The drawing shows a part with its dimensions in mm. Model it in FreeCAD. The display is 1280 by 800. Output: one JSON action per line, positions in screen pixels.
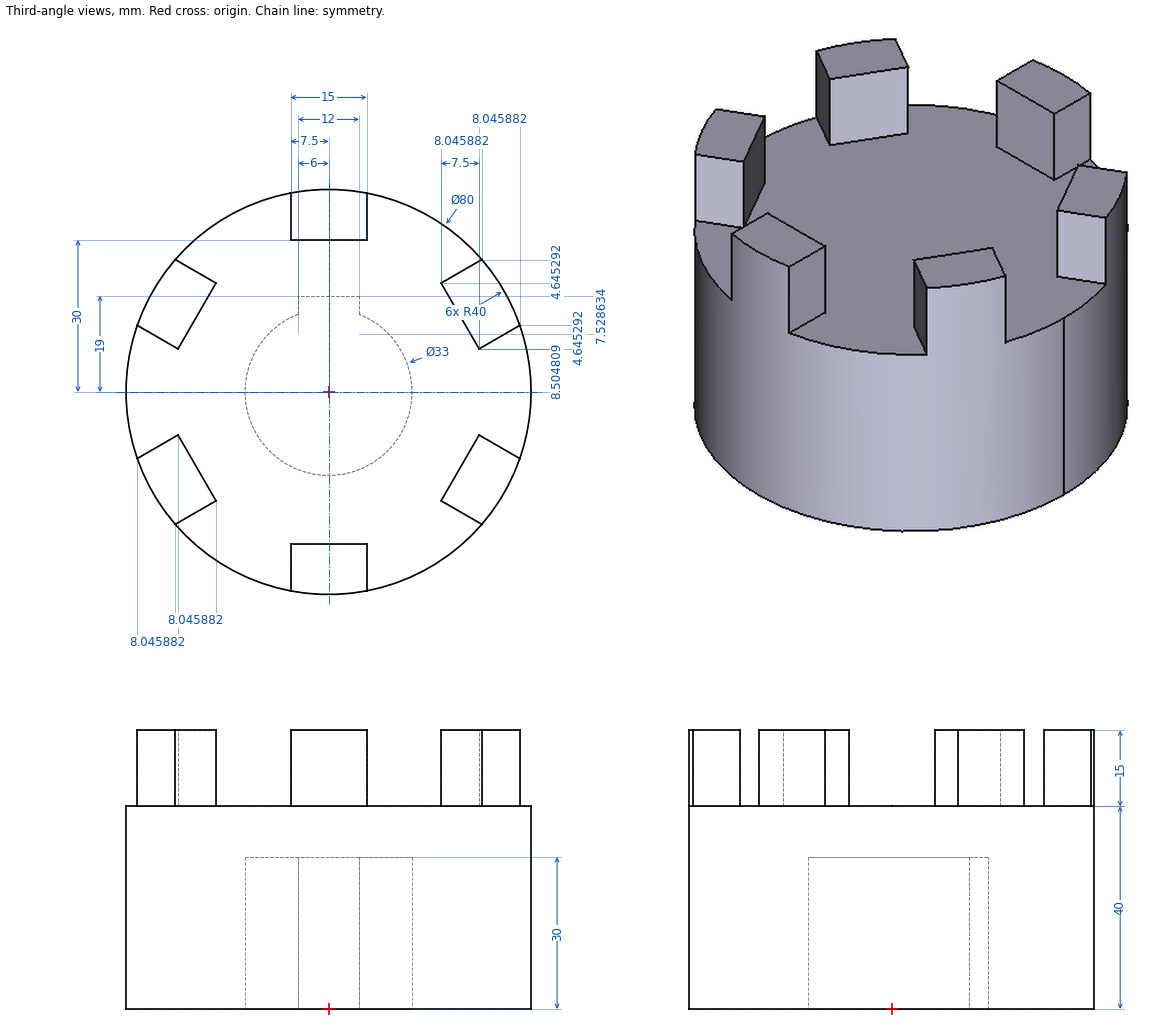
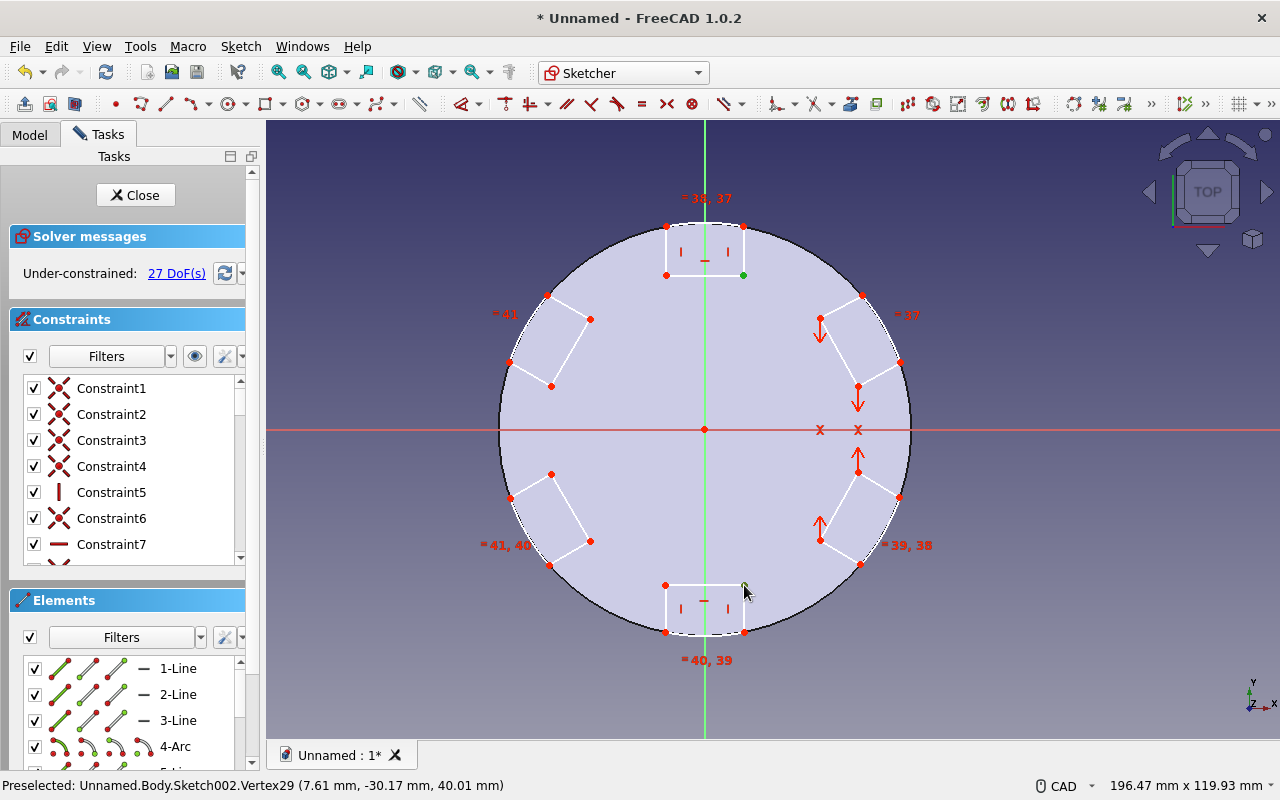
{"action": "left_click", "coordinate": [353, 429]}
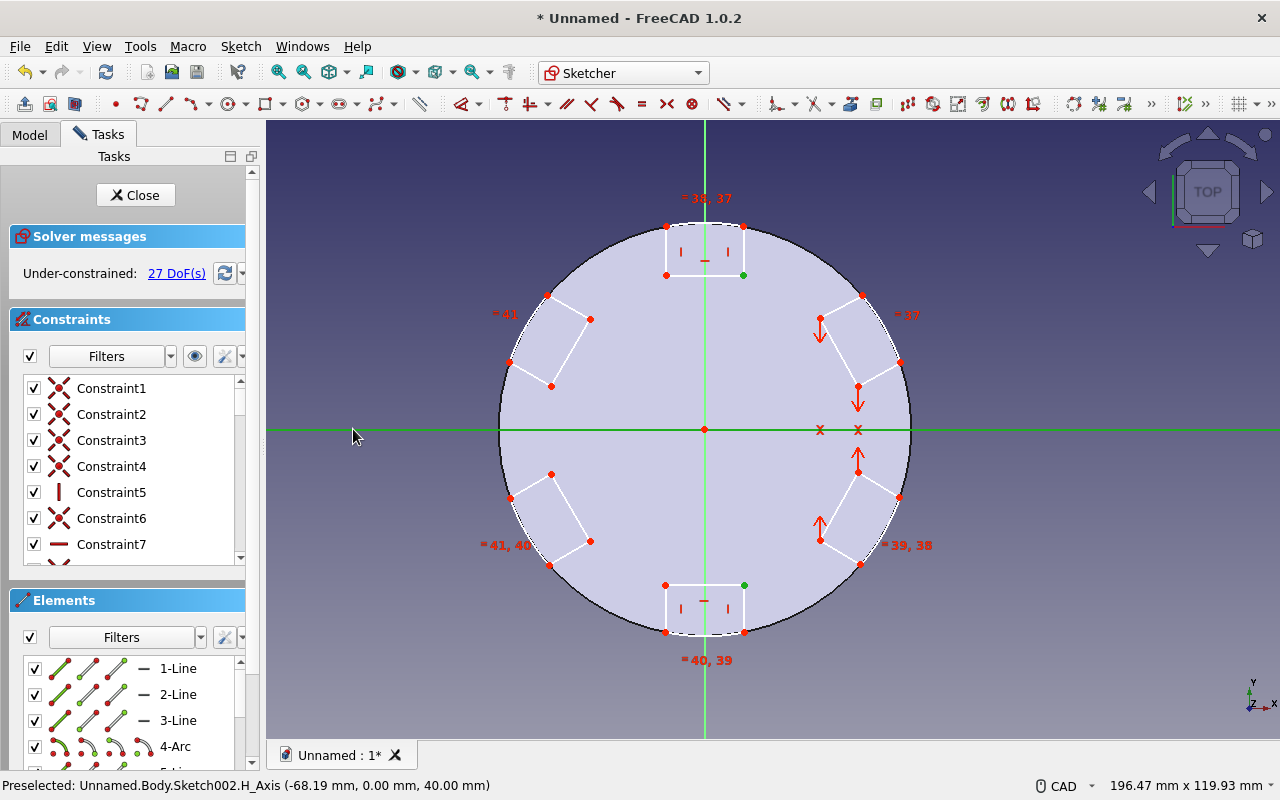
{"action": "key", "text": "s"}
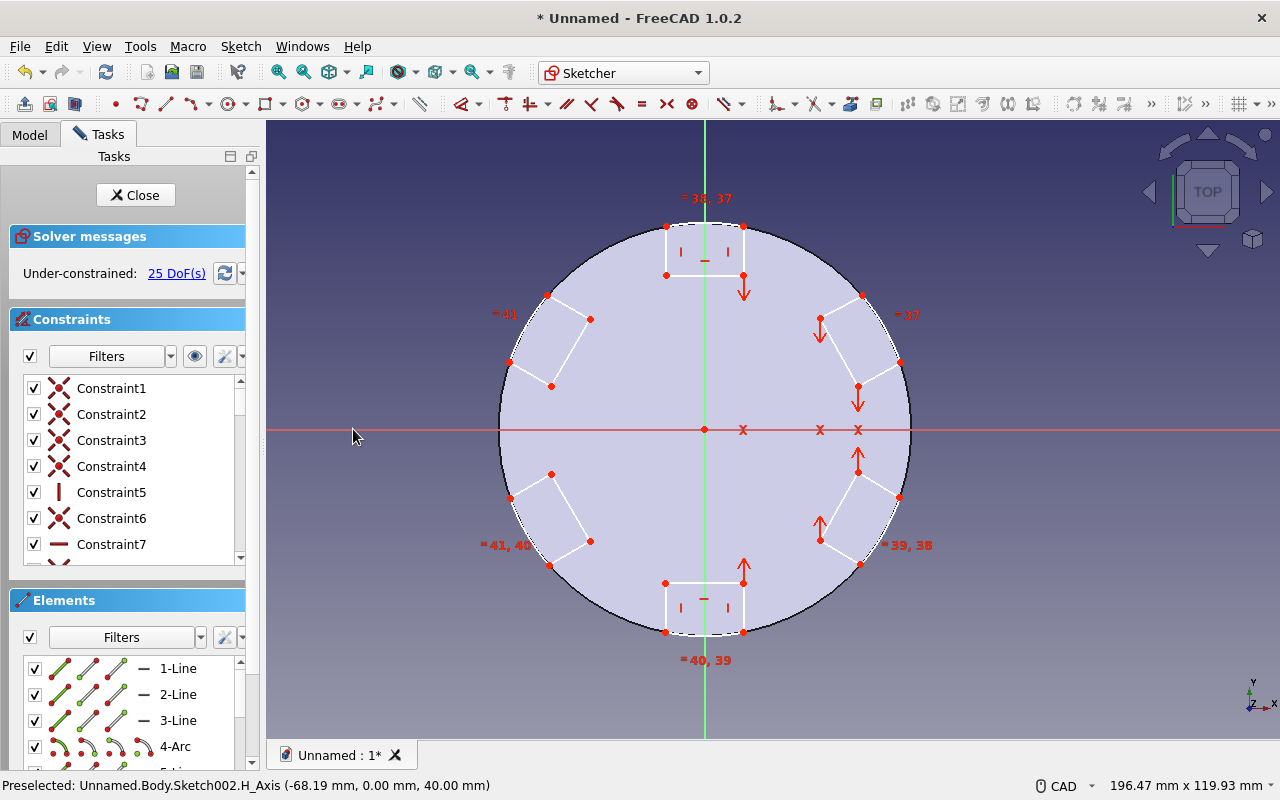
{"action": "left_click", "coordinate": [820, 541]}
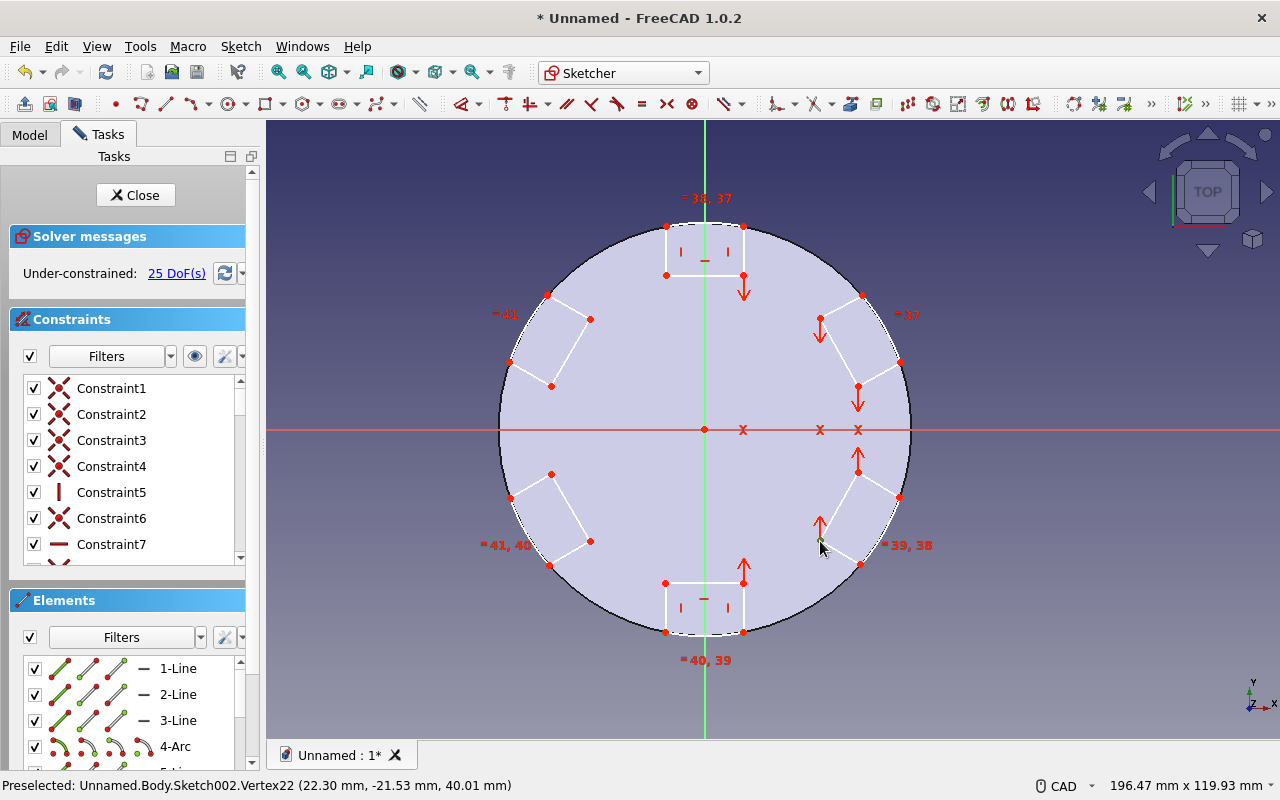
{"action": "left_click", "coordinate": [590, 541]}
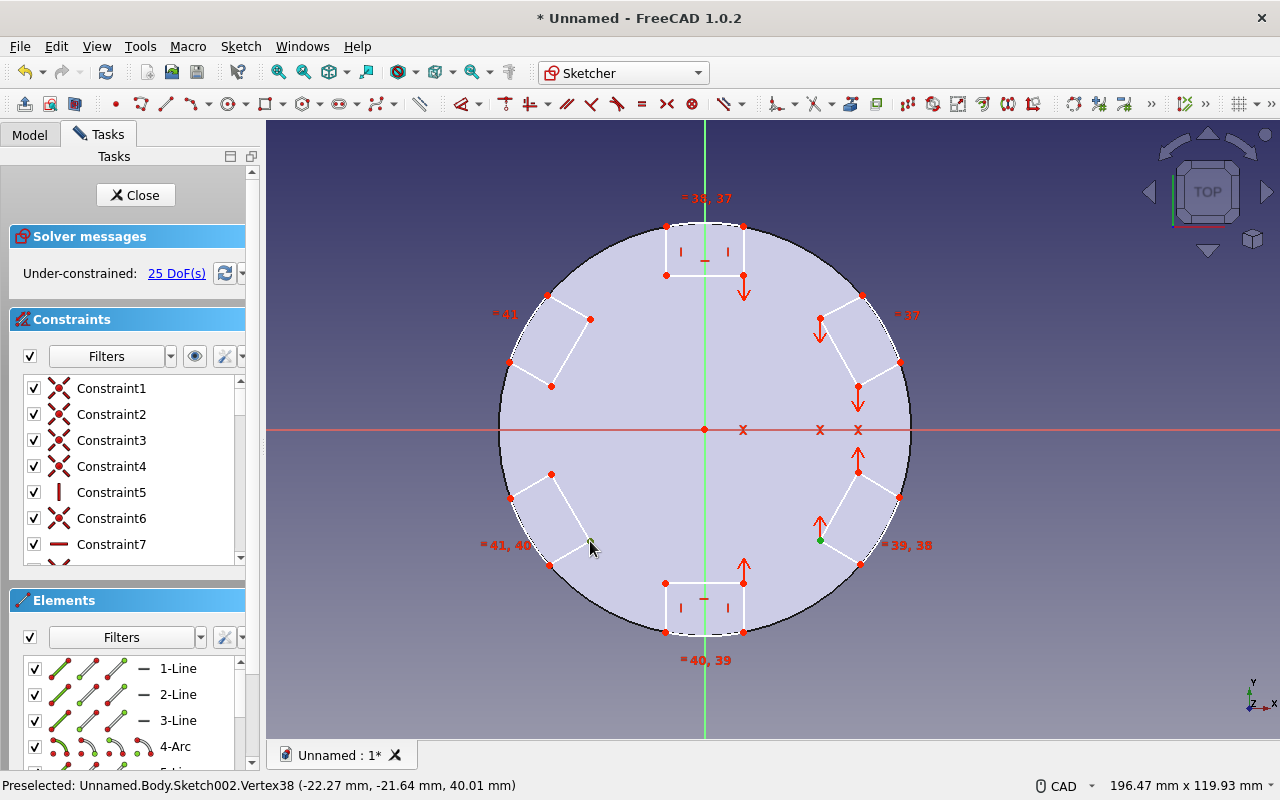
{"action": "left_click", "coordinate": [705, 671]}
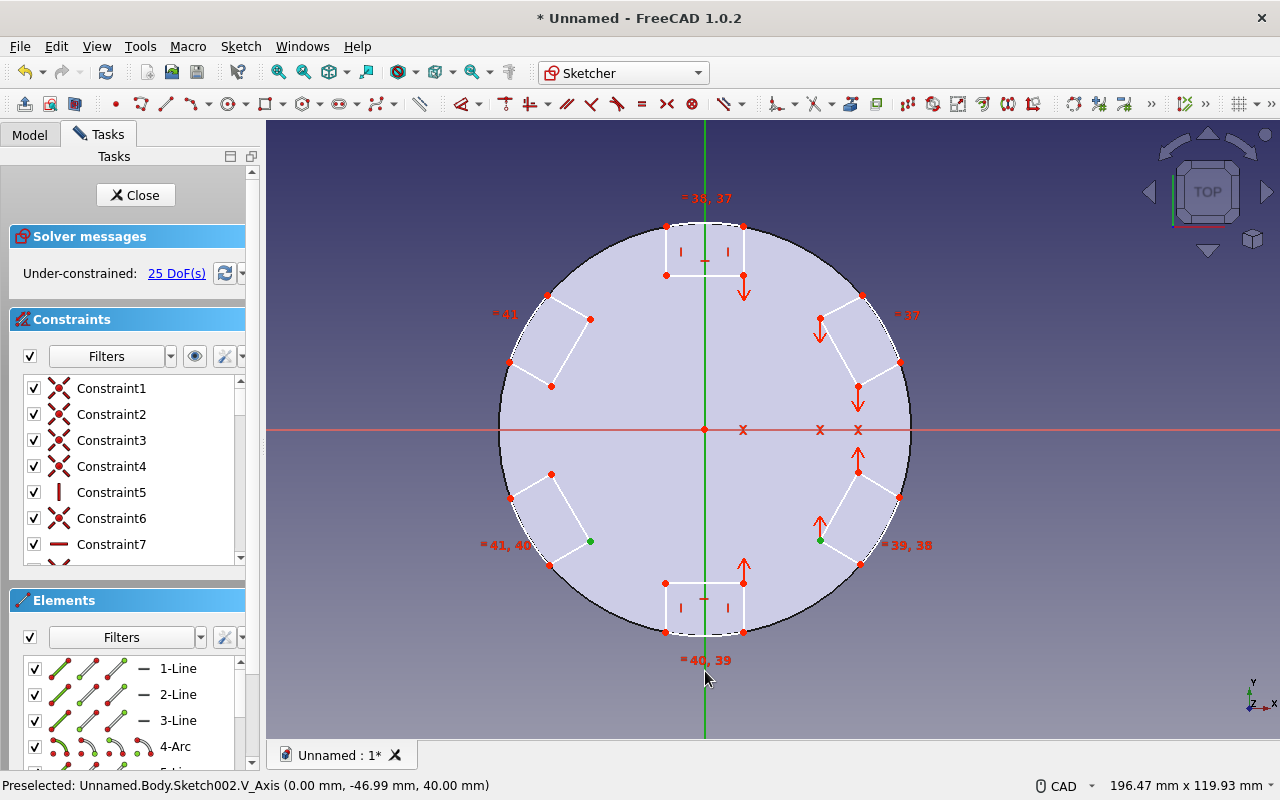
{"action": "key", "text": "s"}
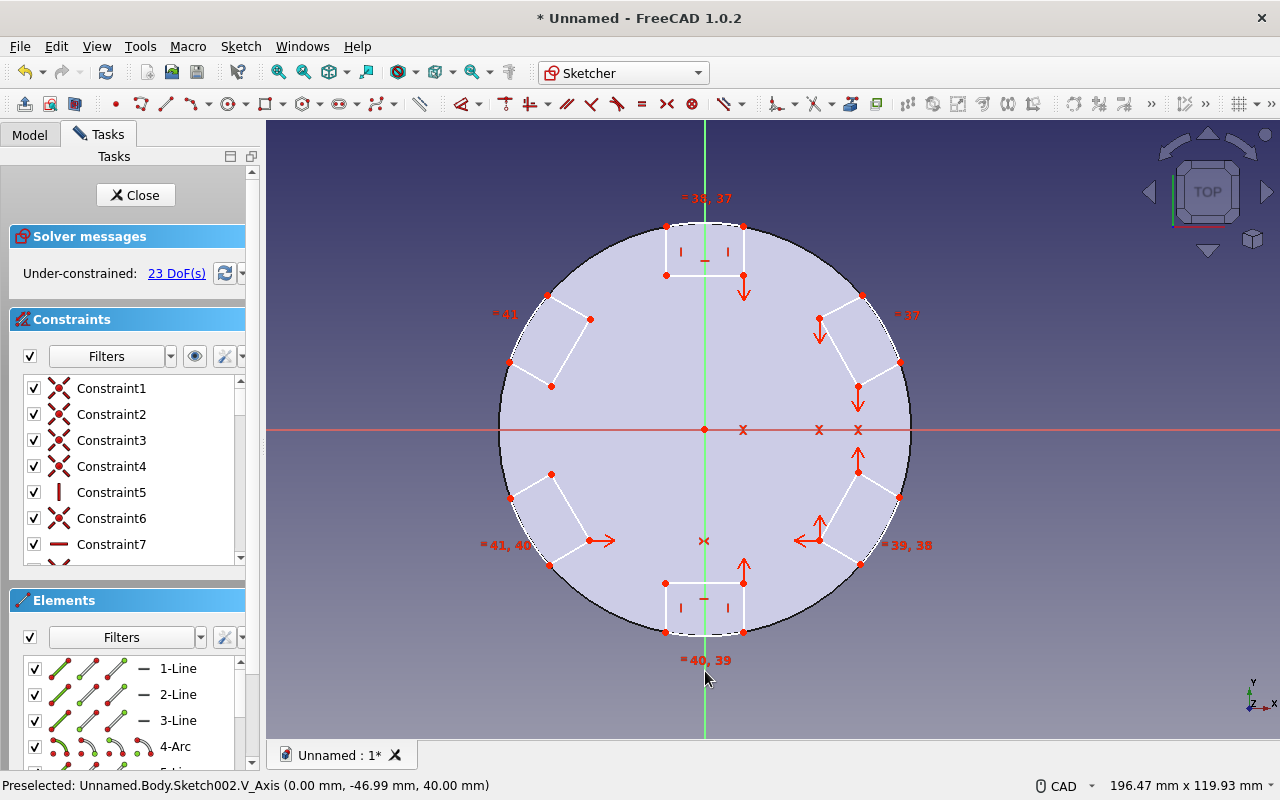
{"action": "left_click", "coordinate": [858, 472]}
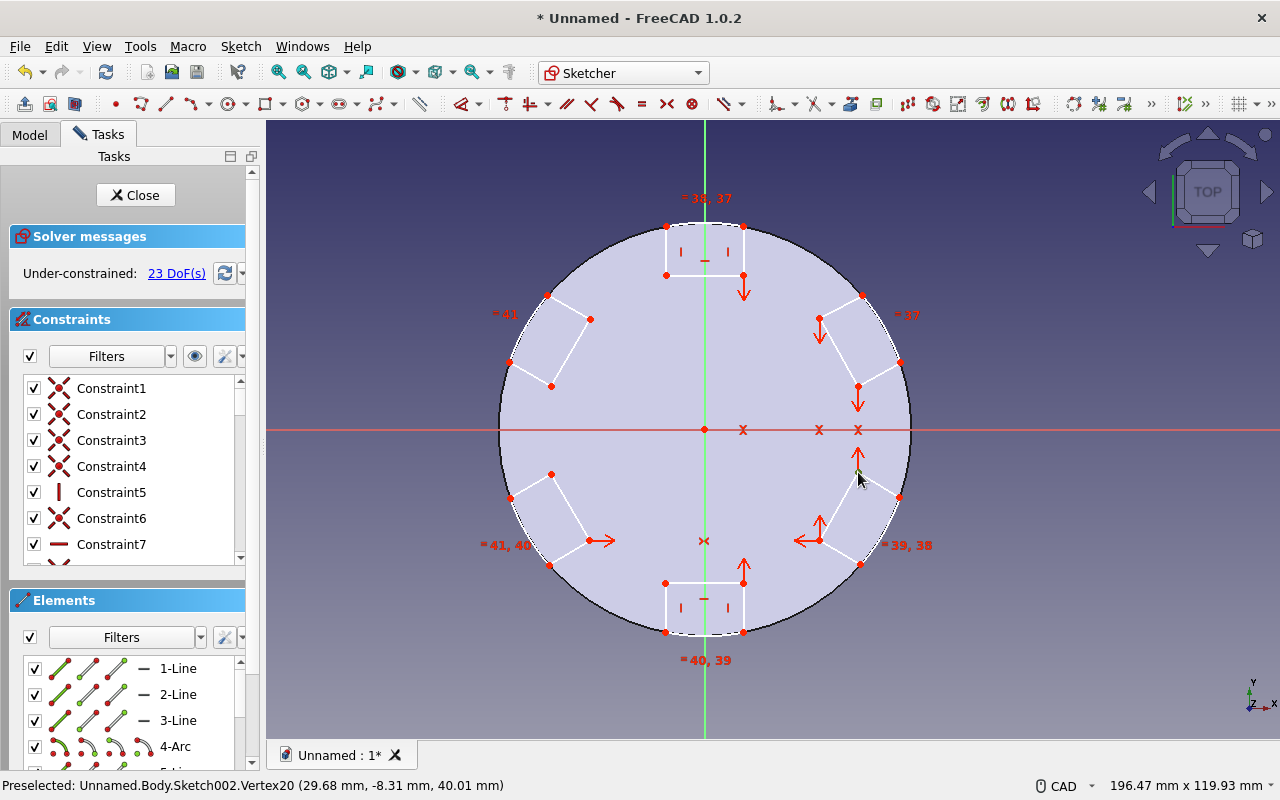
{"action": "left_click", "coordinate": [551, 474]}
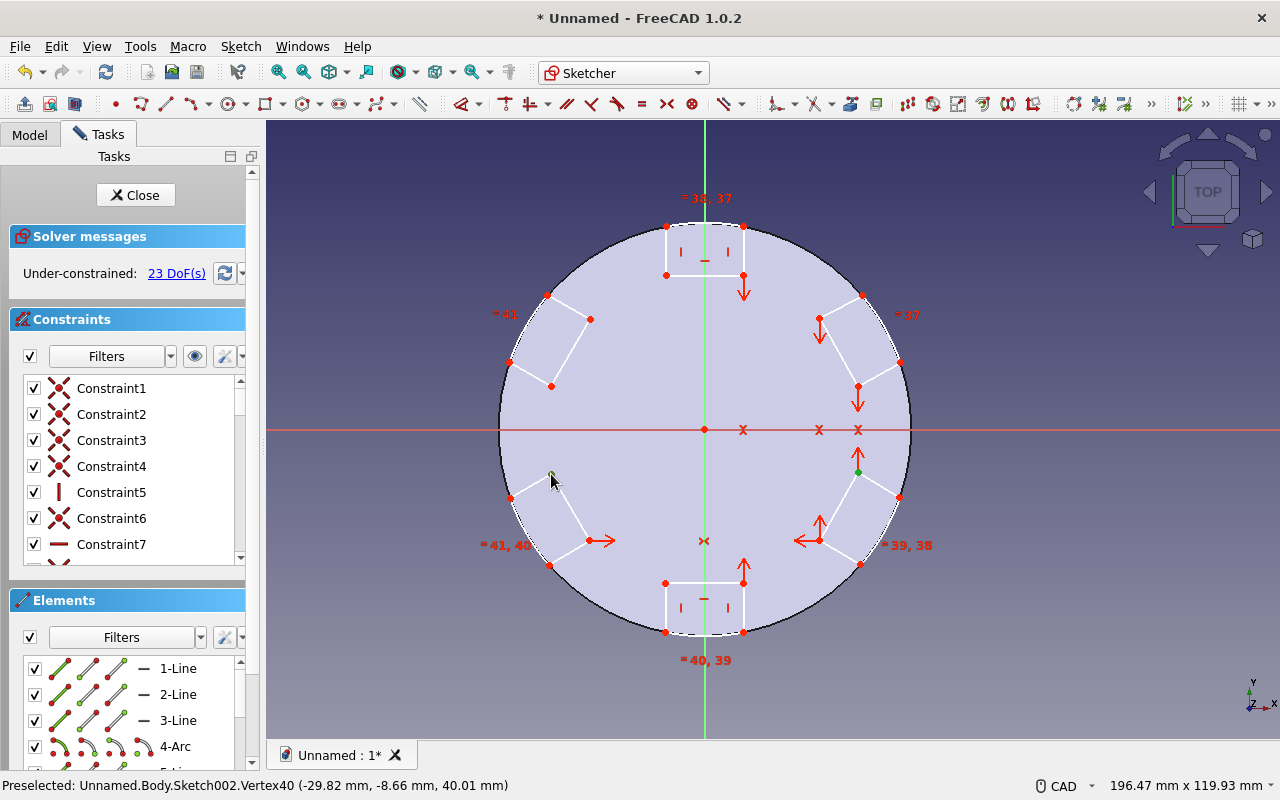
{"action": "left_click", "coordinate": [705, 671]}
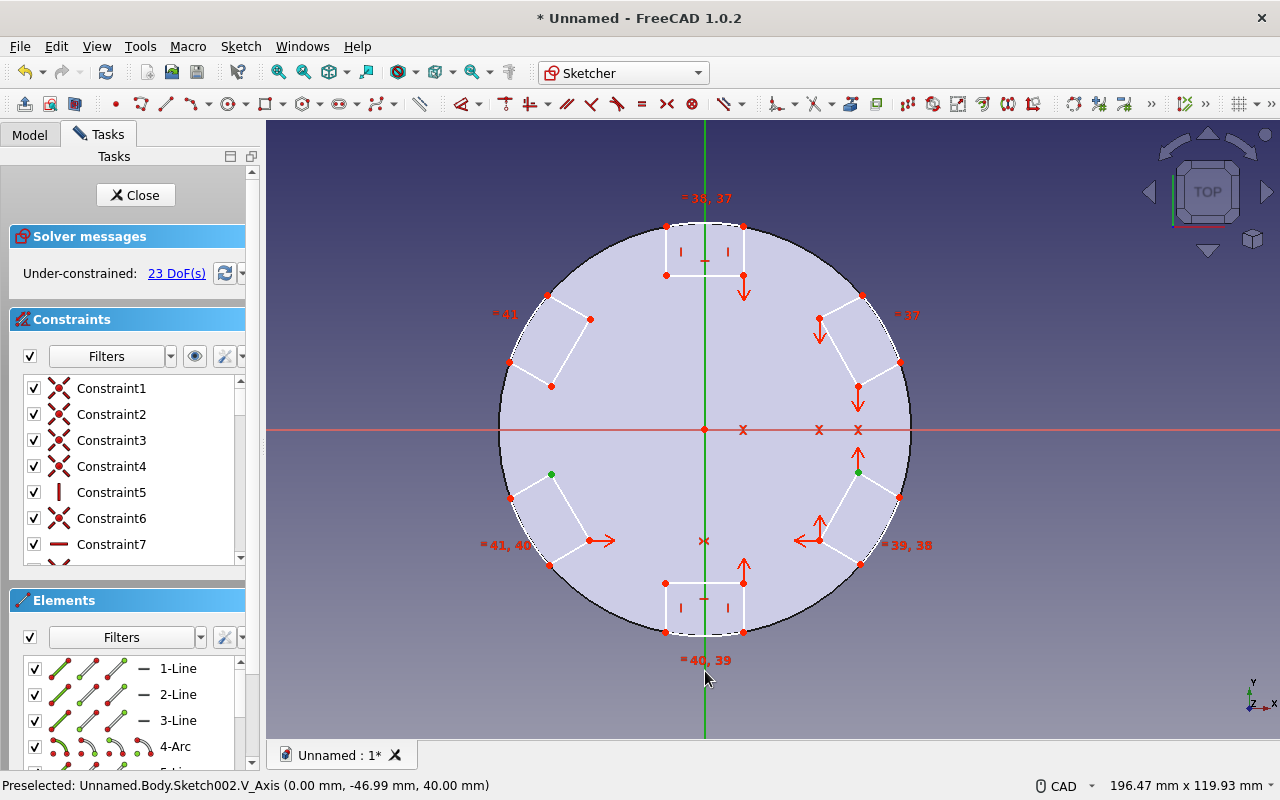
{"action": "key", "text": "s"}